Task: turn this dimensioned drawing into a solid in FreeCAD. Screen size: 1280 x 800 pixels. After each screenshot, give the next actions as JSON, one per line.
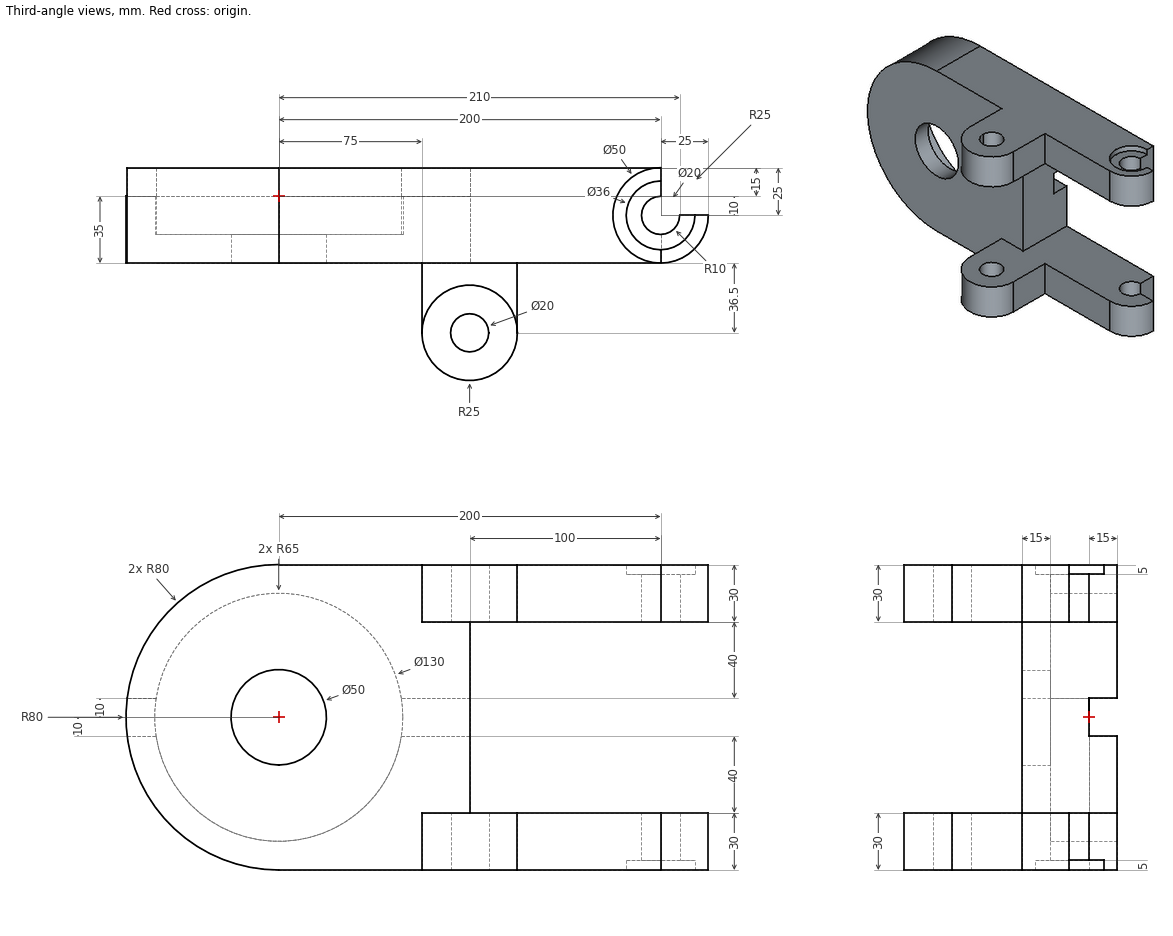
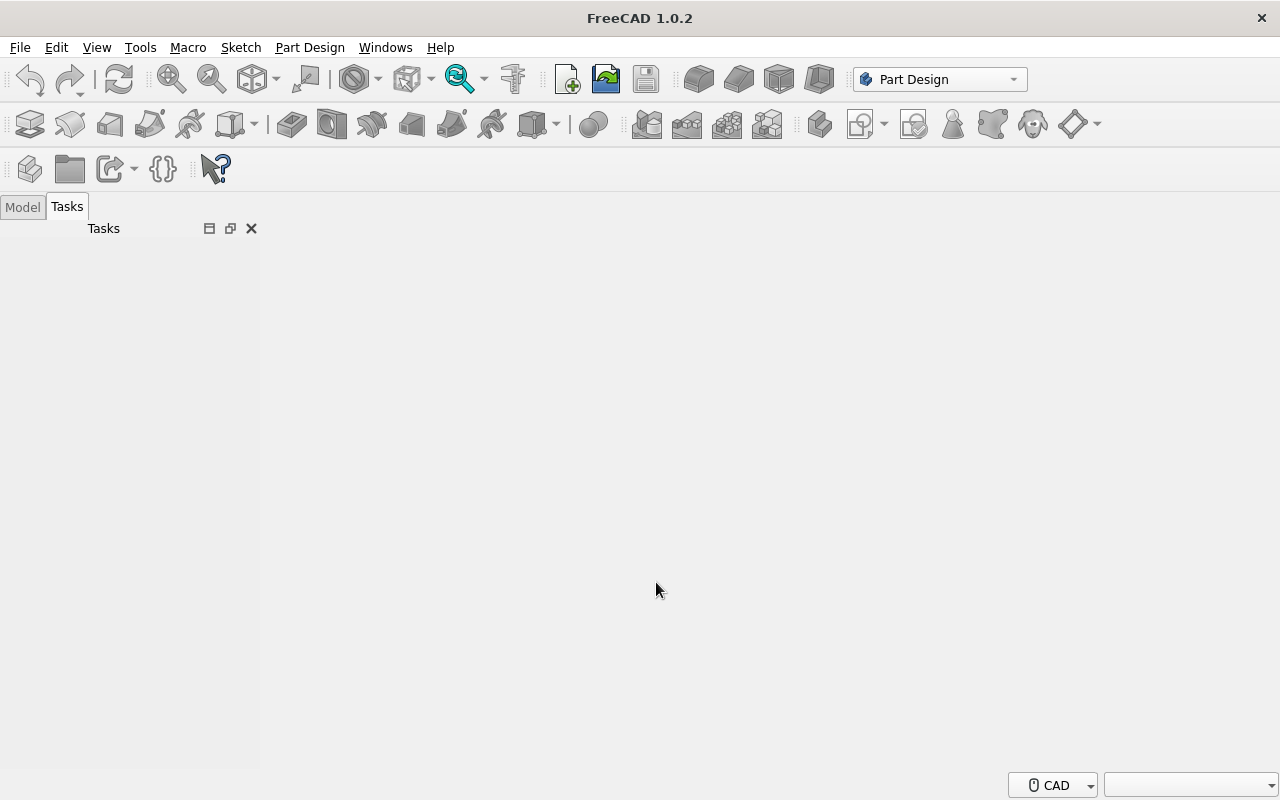
{"action": "left_click", "coordinate": [566, 80]}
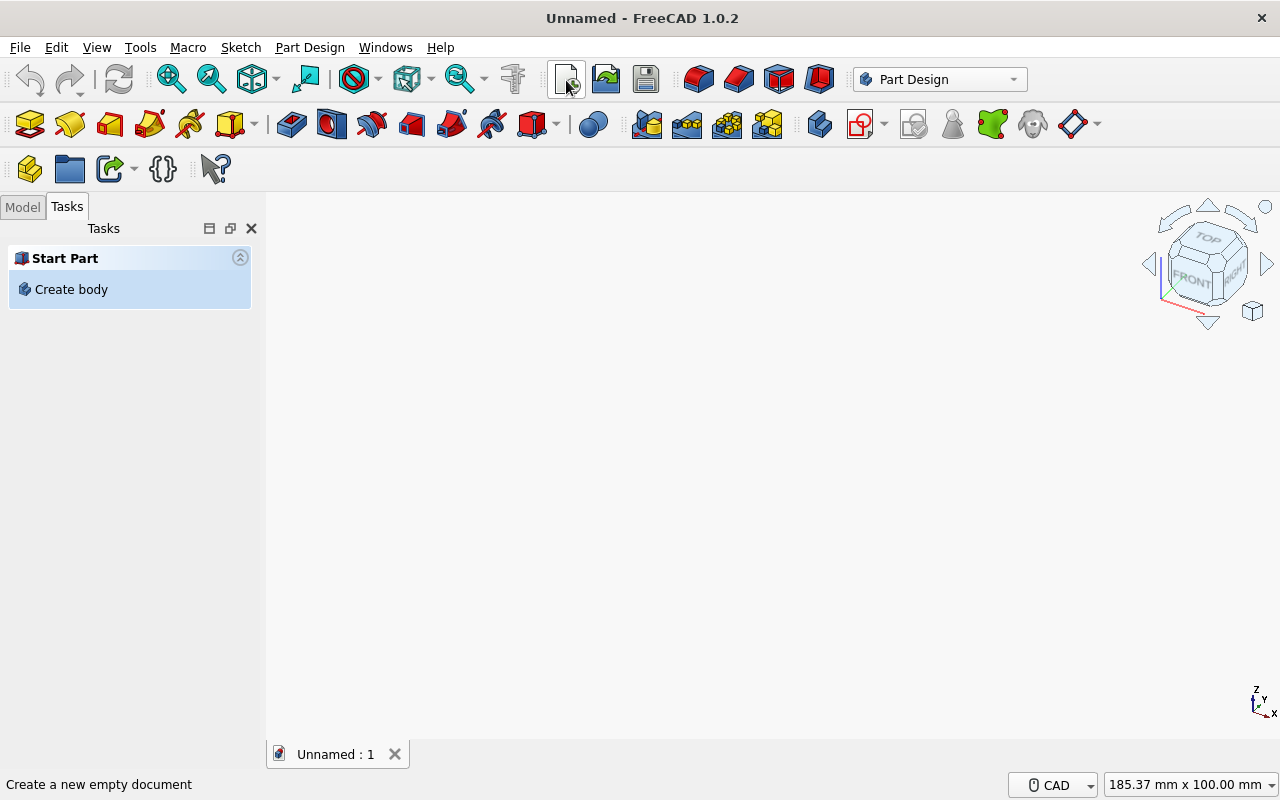
{"action": "left_click", "coordinate": [820, 124]}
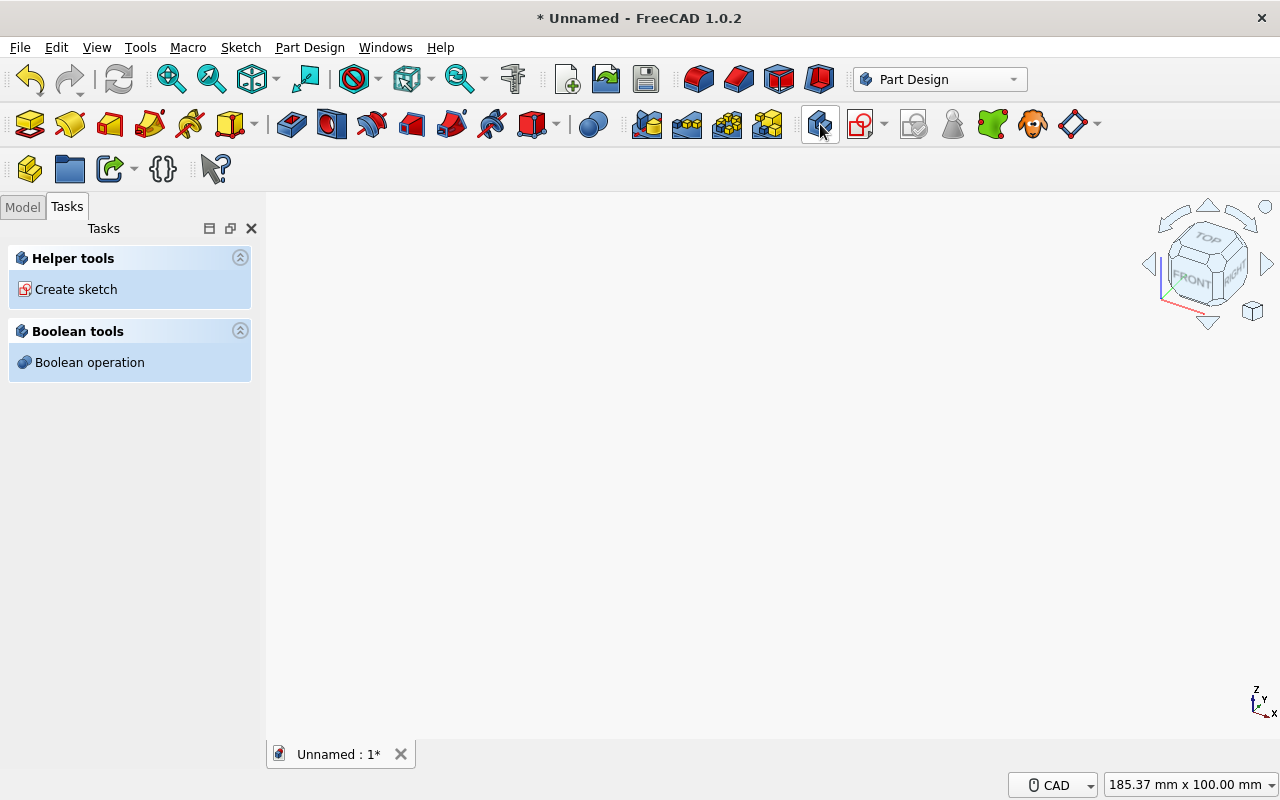
{"action": "left_click", "coordinate": [23, 206]}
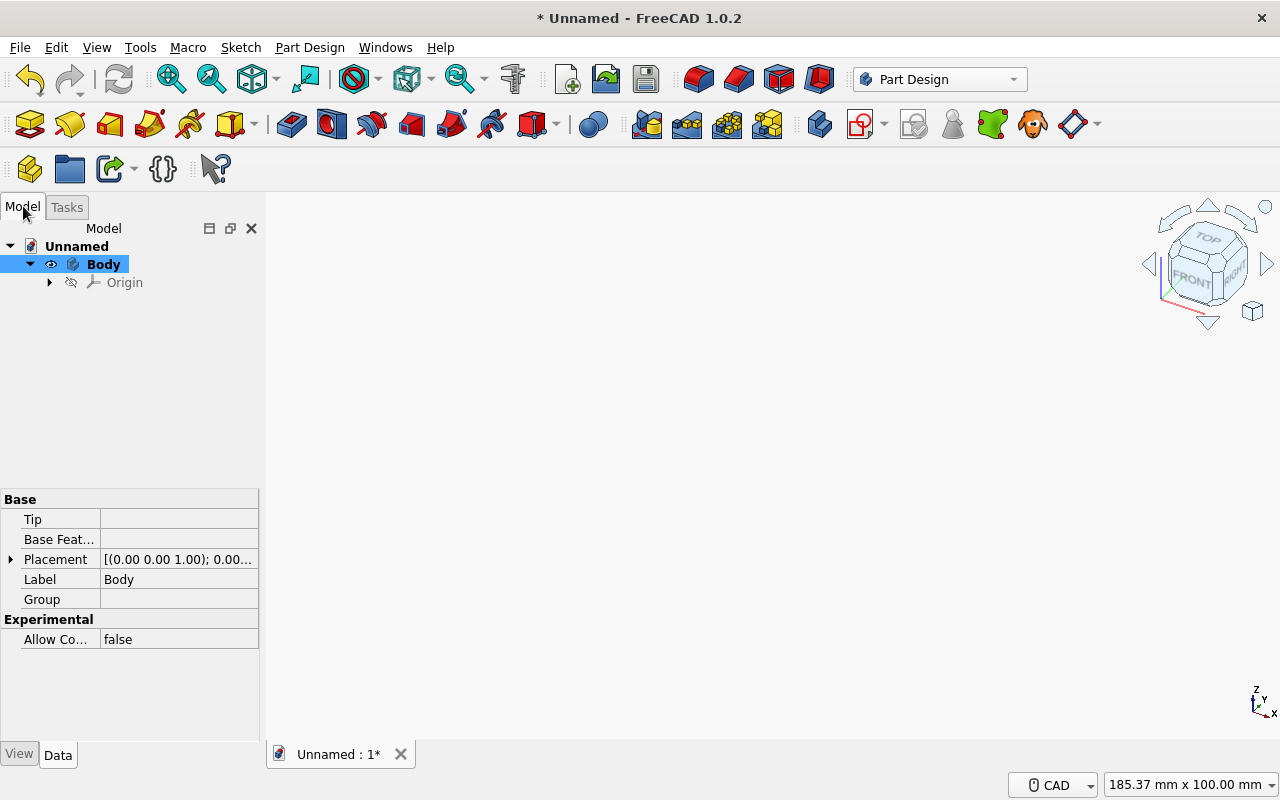
{"action": "left_click", "coordinate": [96, 264]}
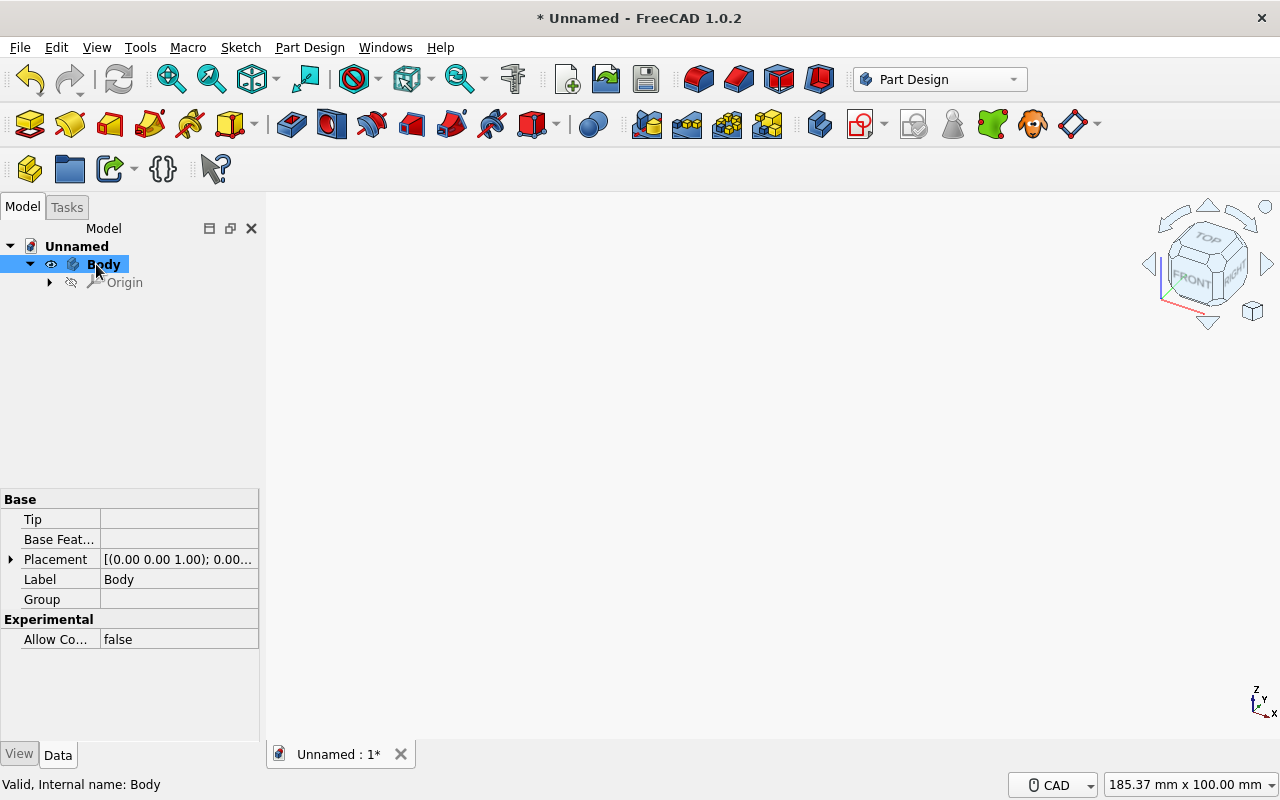
{"action": "left_click", "coordinate": [146, 639]}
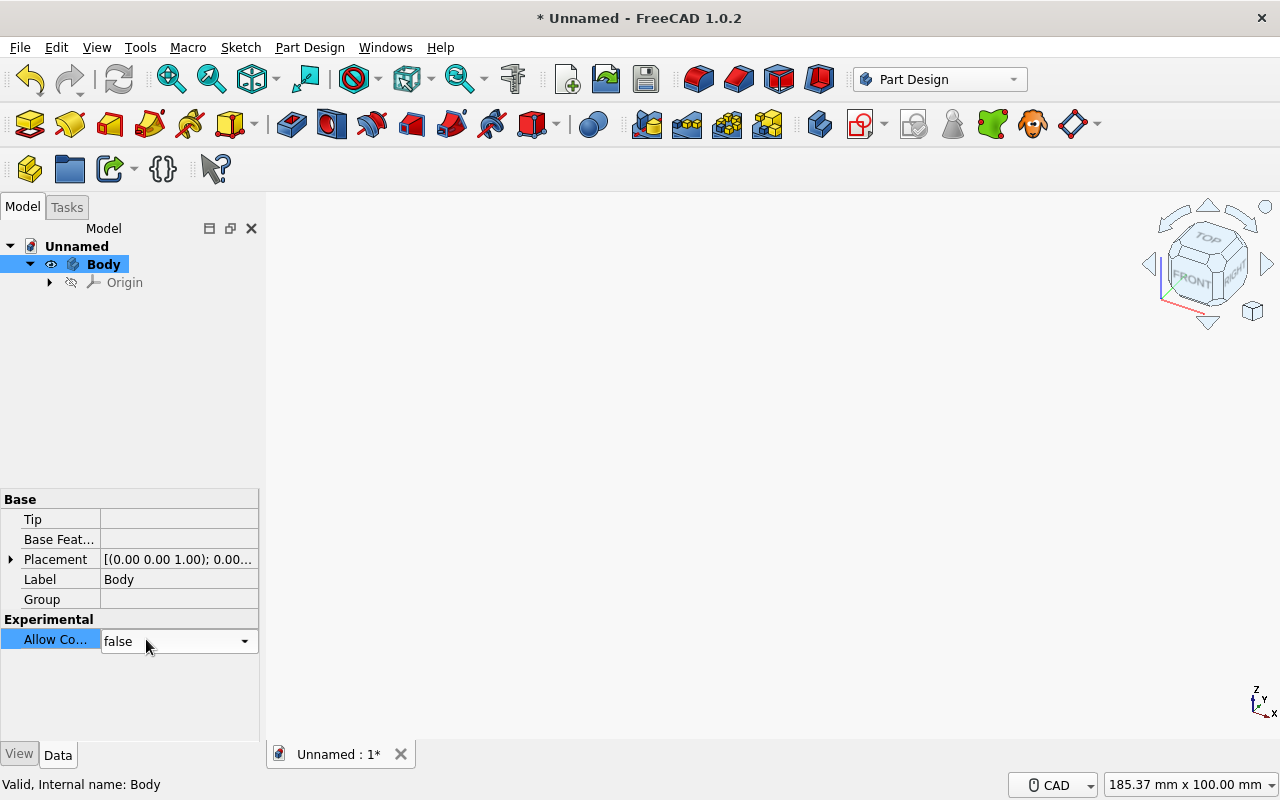
{"action": "left_click", "coordinate": [146, 639]}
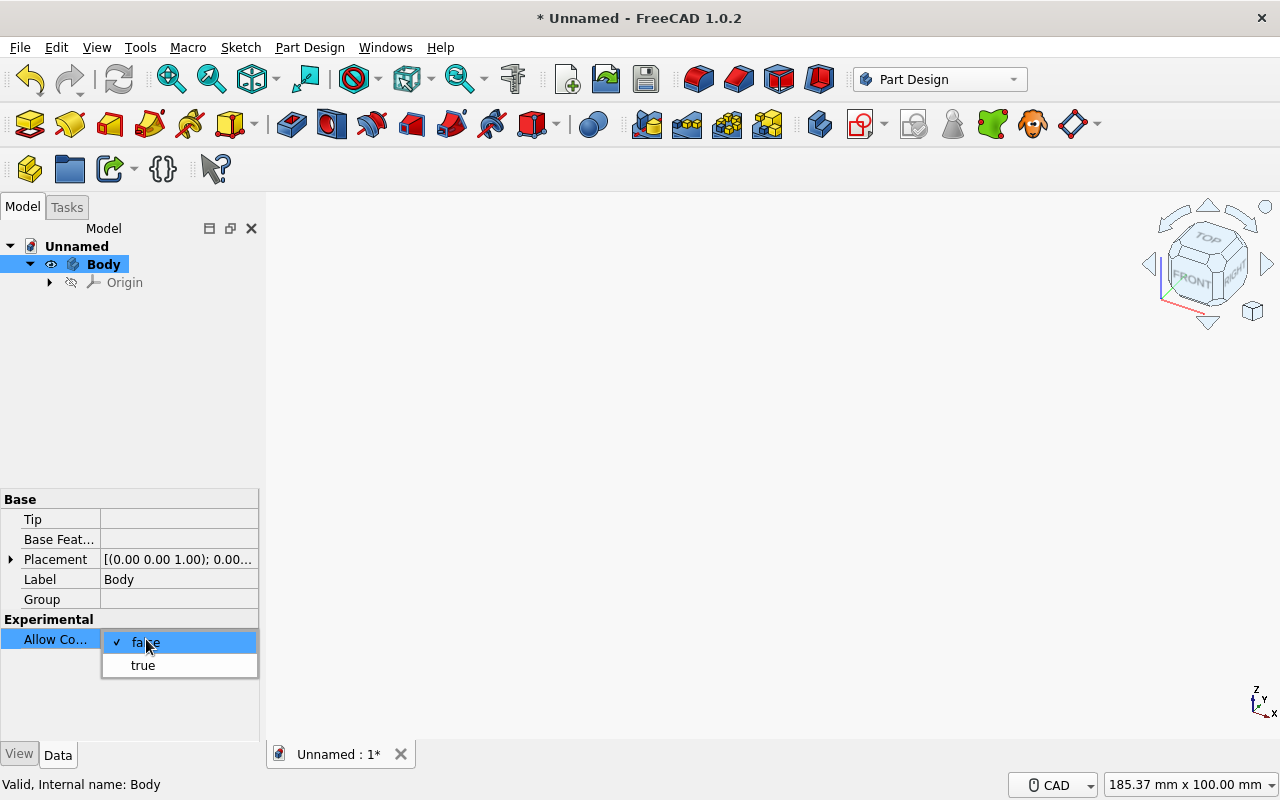
{"action": "left_click", "coordinate": [179, 666]}
{"action": "key", "text": "Return"}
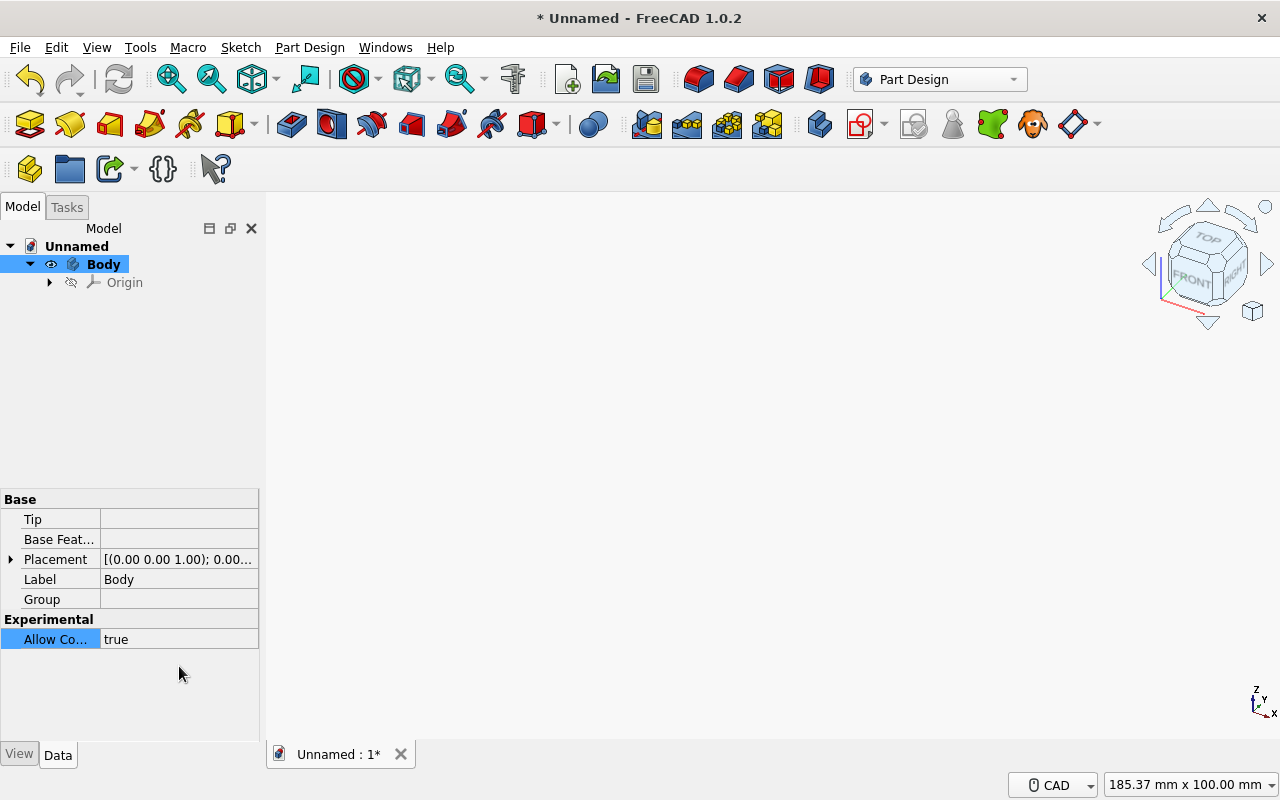
{"action": "left_click", "coordinate": [306, 699]}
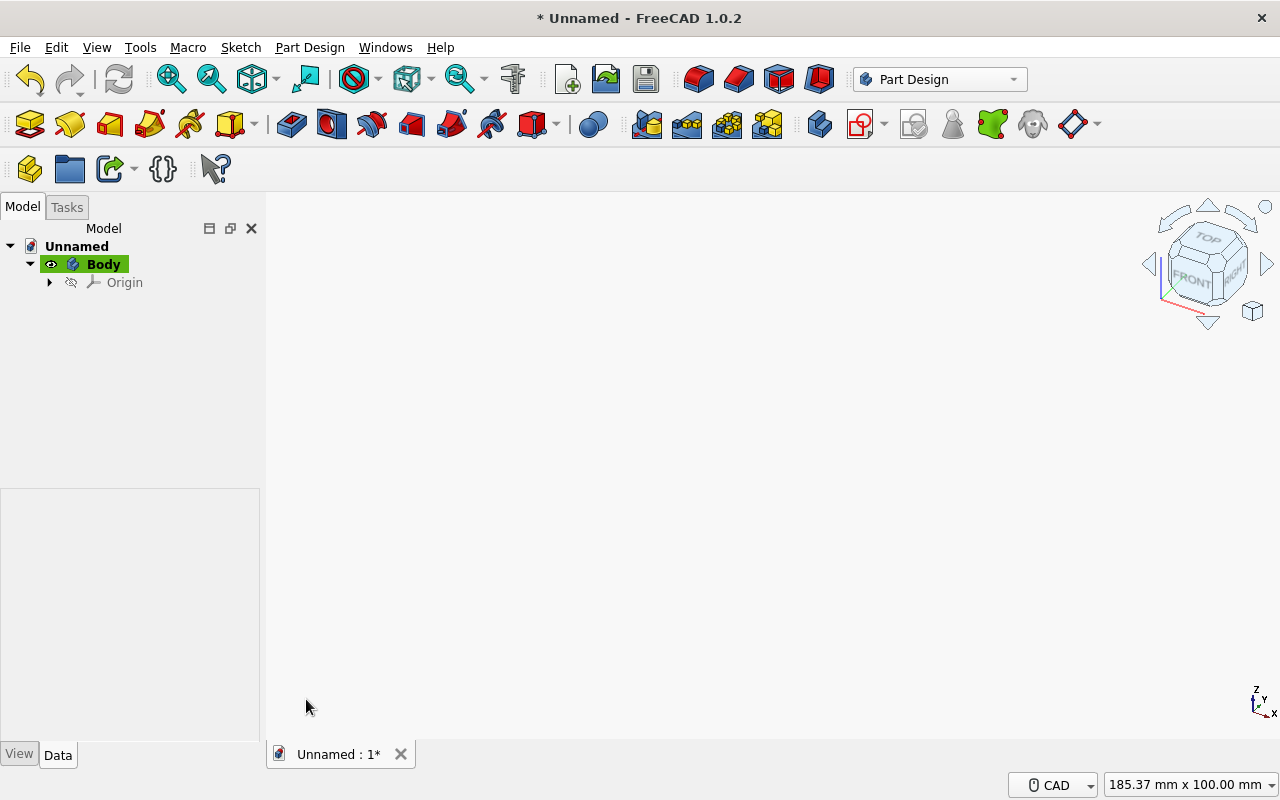
{"action": "left_click", "coordinate": [860, 124]}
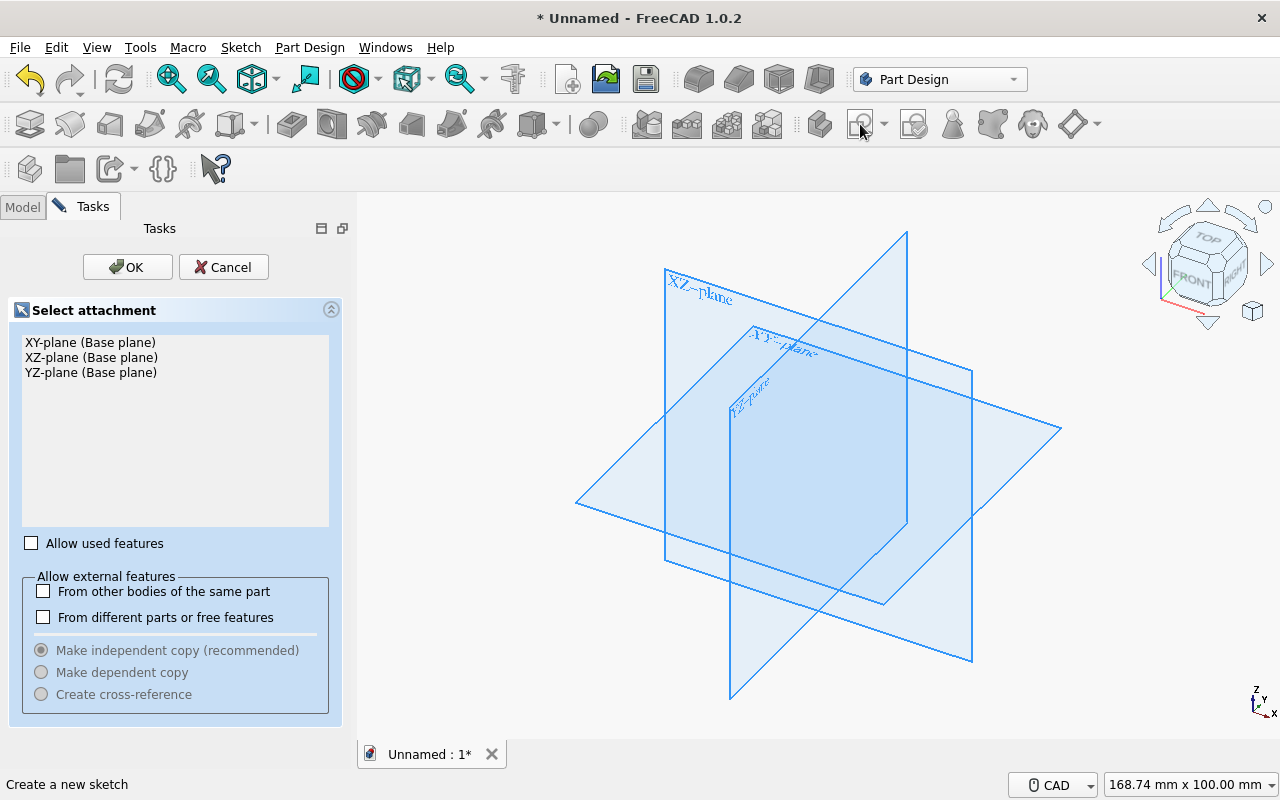
{"action": "left_click", "coordinate": [82, 358]}